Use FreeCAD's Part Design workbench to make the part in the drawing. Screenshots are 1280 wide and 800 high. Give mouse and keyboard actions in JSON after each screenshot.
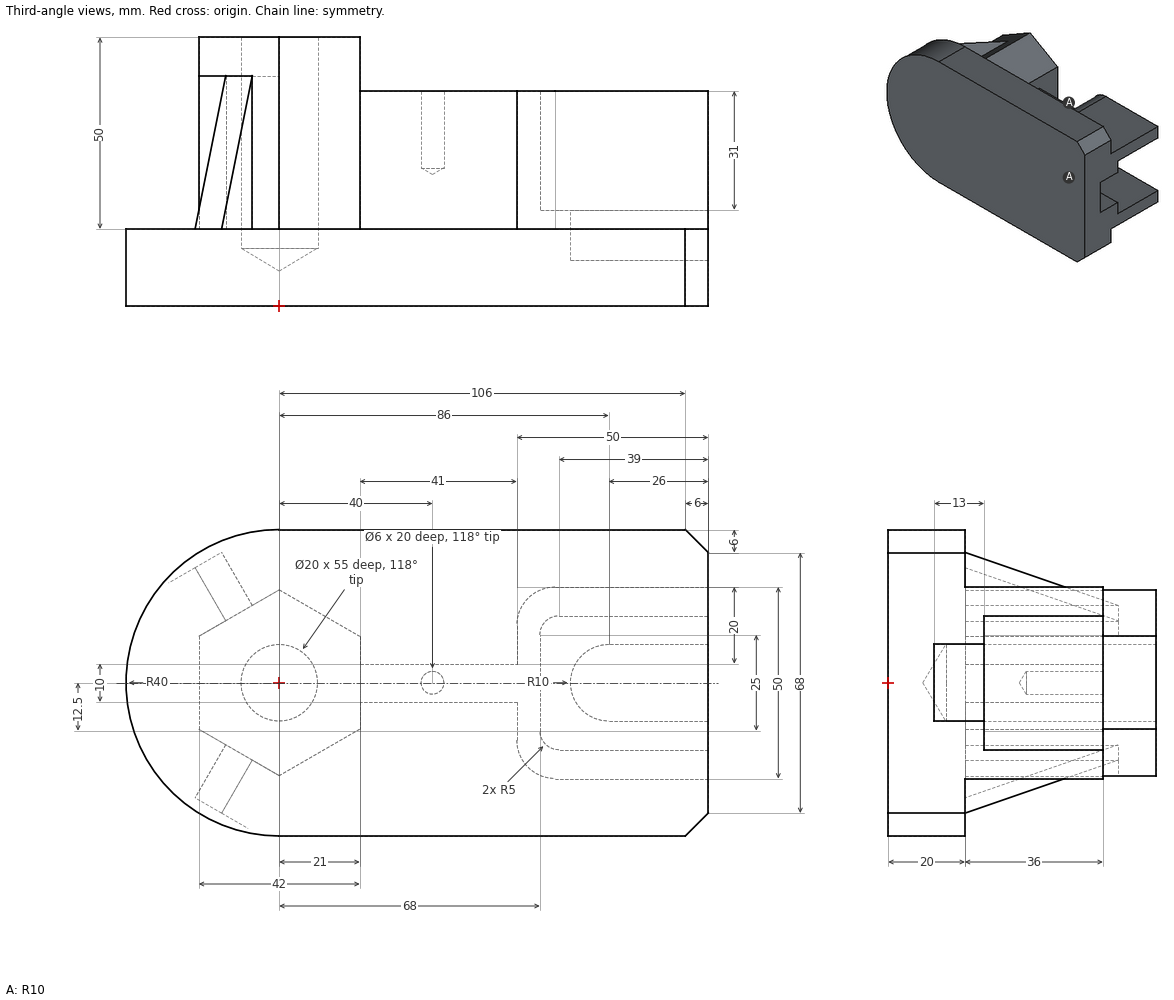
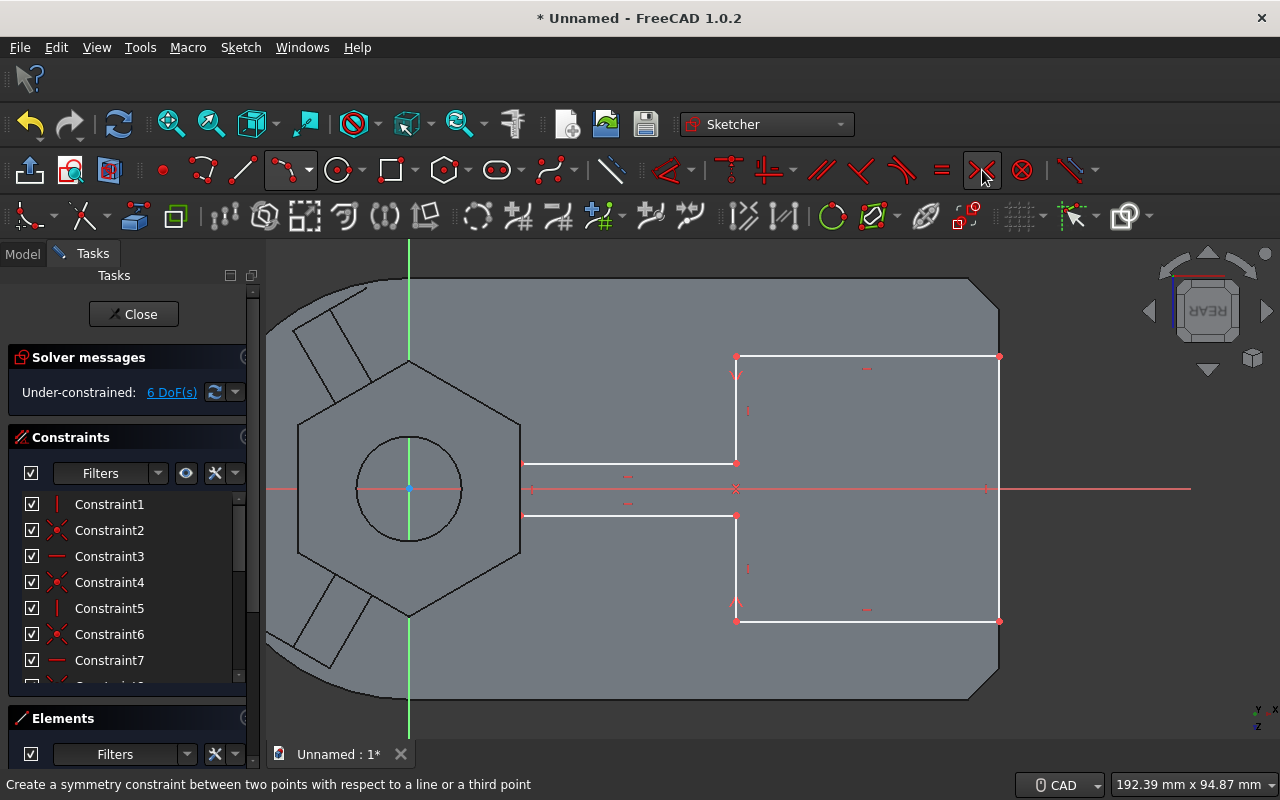
{"action": "left_click", "coordinate": [666, 170]}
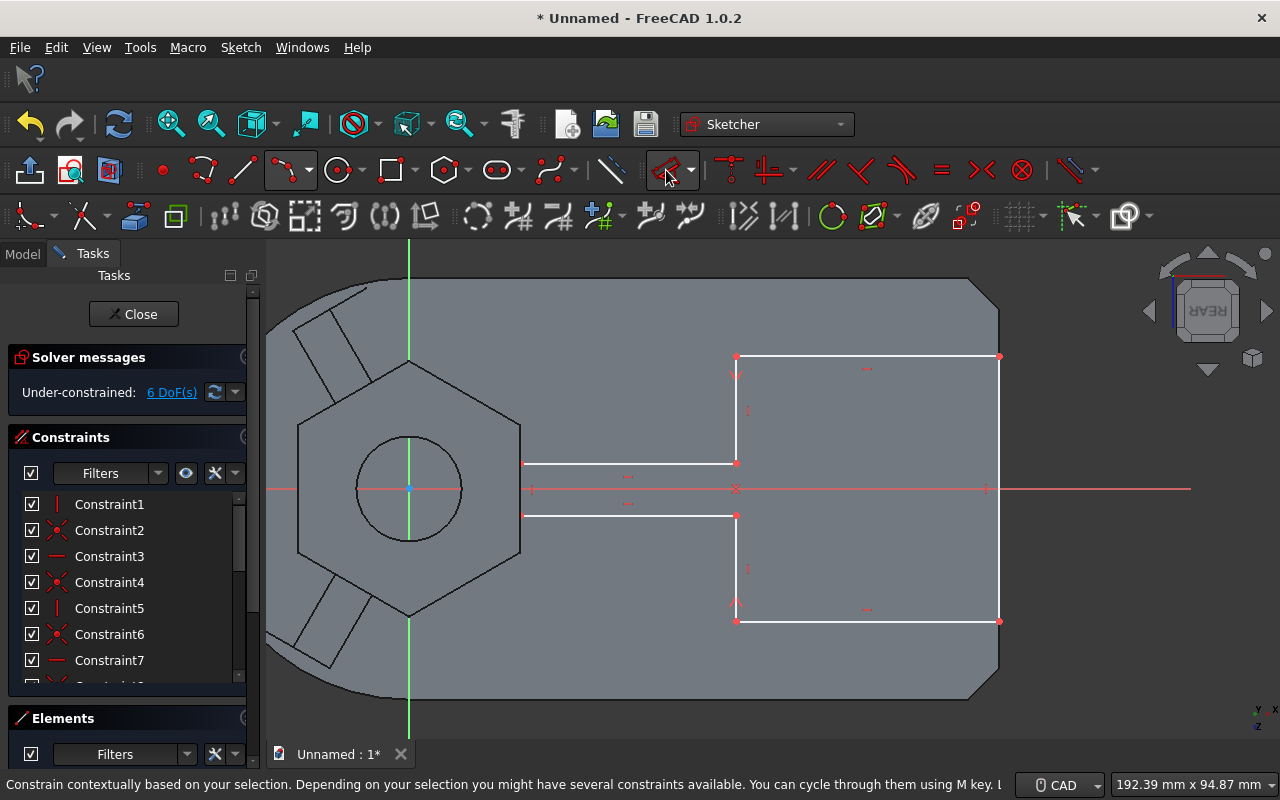
{"action": "scroll", "coordinate": [520, 480], "scroll_direction": "up", "scroll_amount": 2}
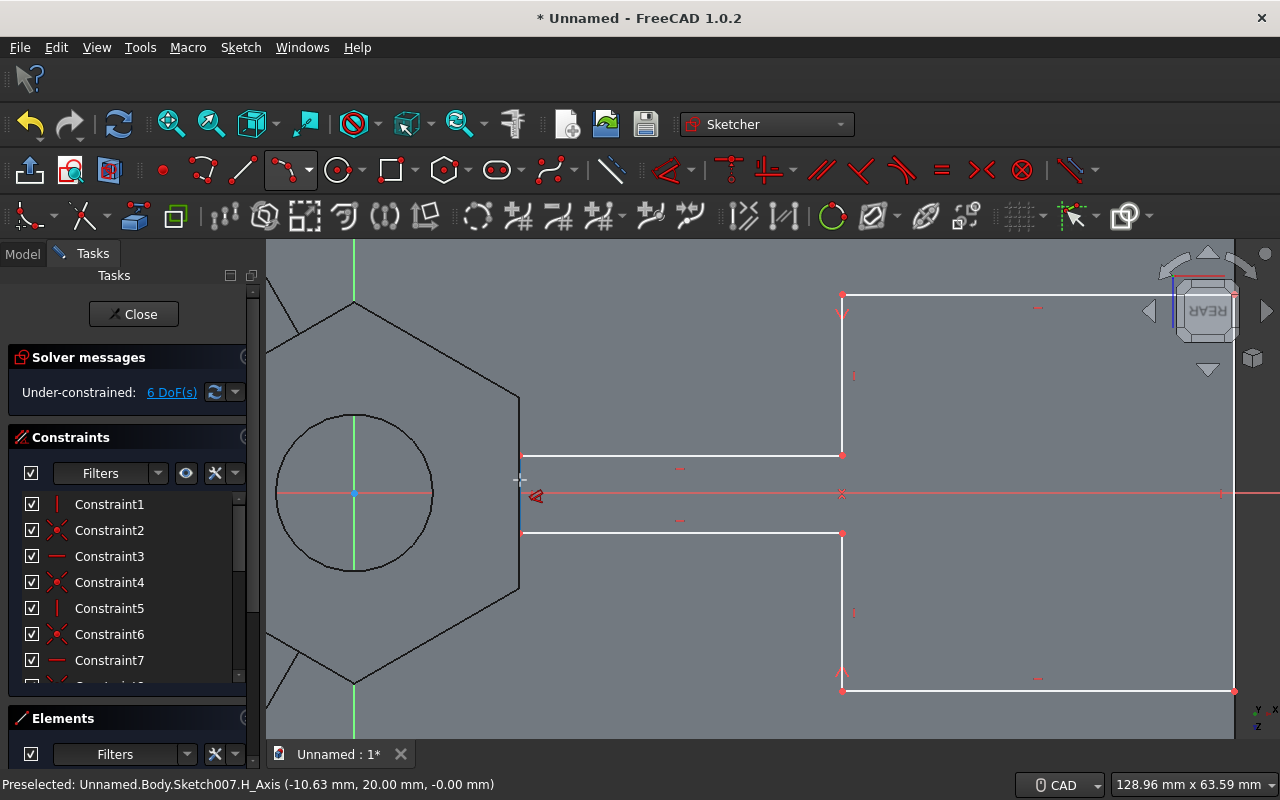
{"action": "left_click", "coordinate": [520, 479]}
{"action": "left_click", "coordinate": [486, 477]}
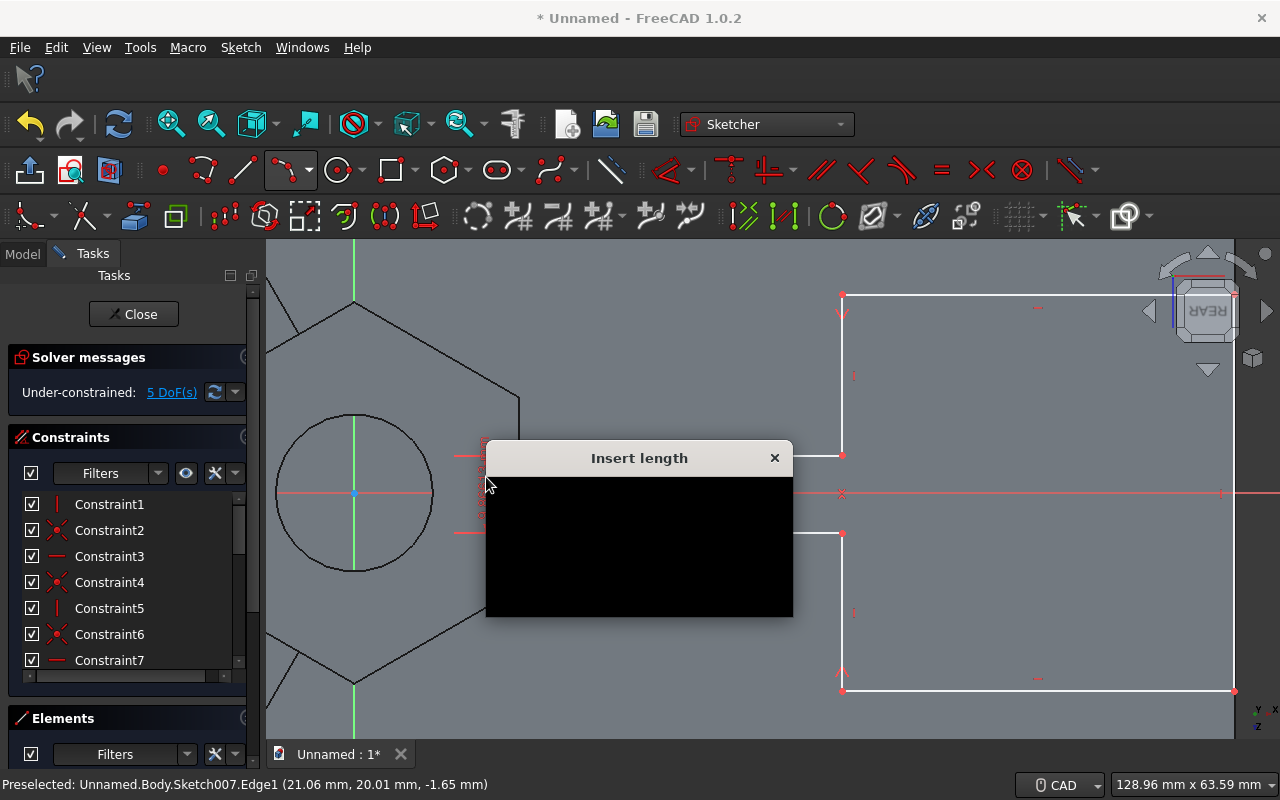
{"action": "type", "text": "10"}
{"action": "key", "text": "Return"}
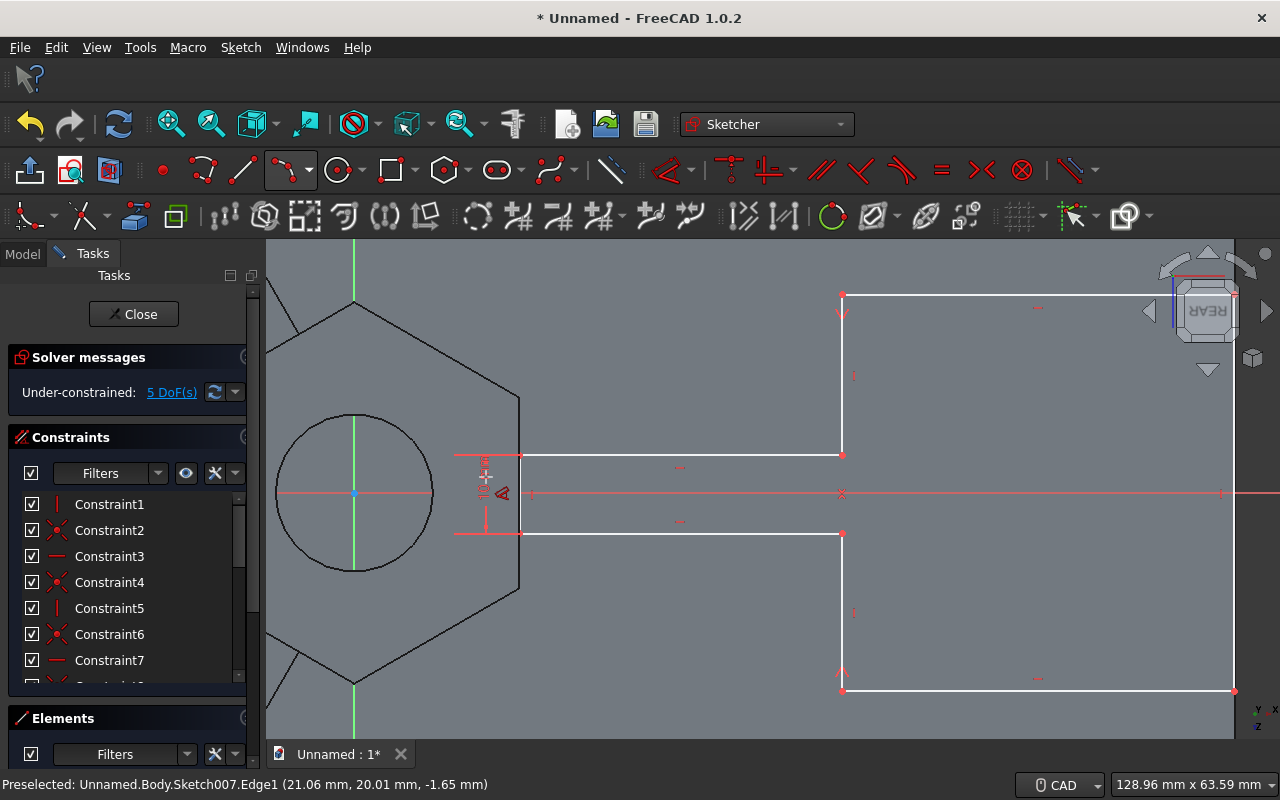
{"action": "left_click", "coordinate": [617, 534]}
{"action": "left_click", "coordinate": [681, 568]}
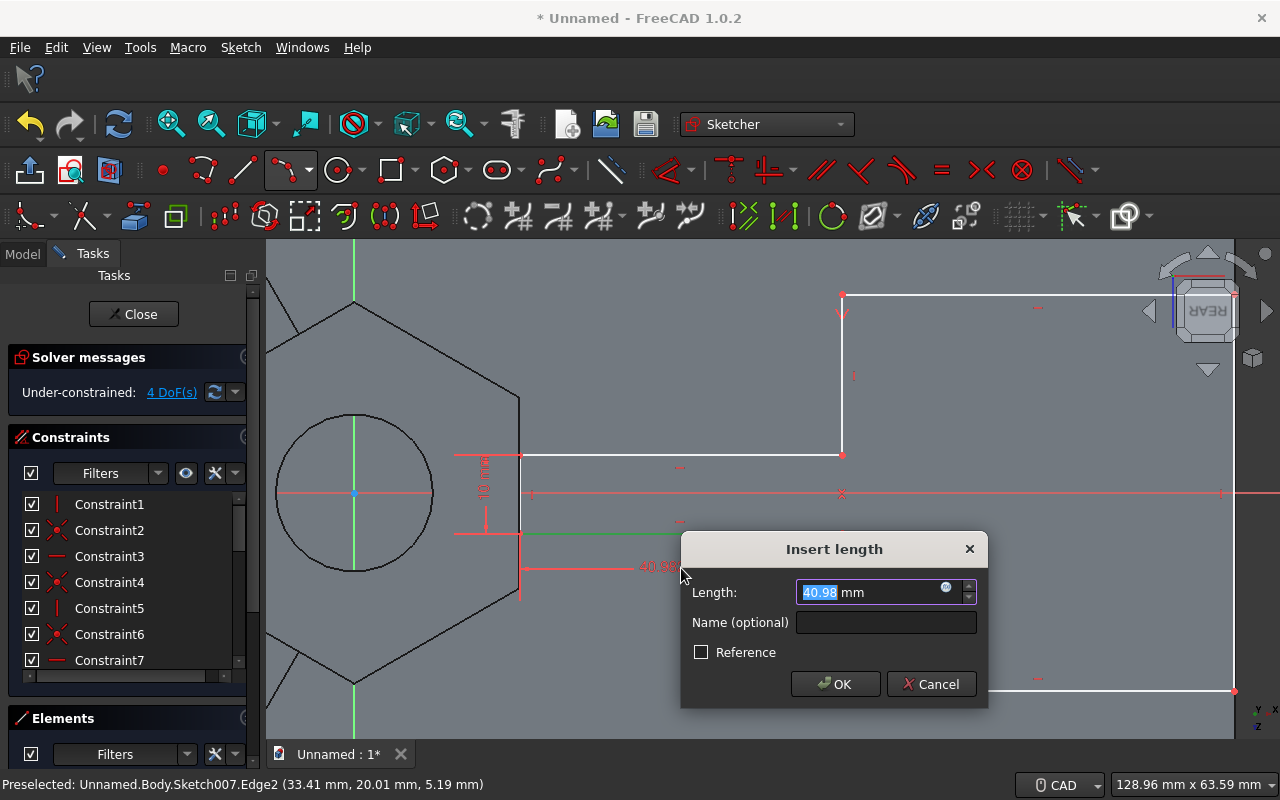
{"action": "type", "text": "41"}
{"action": "key", "text": "Return"}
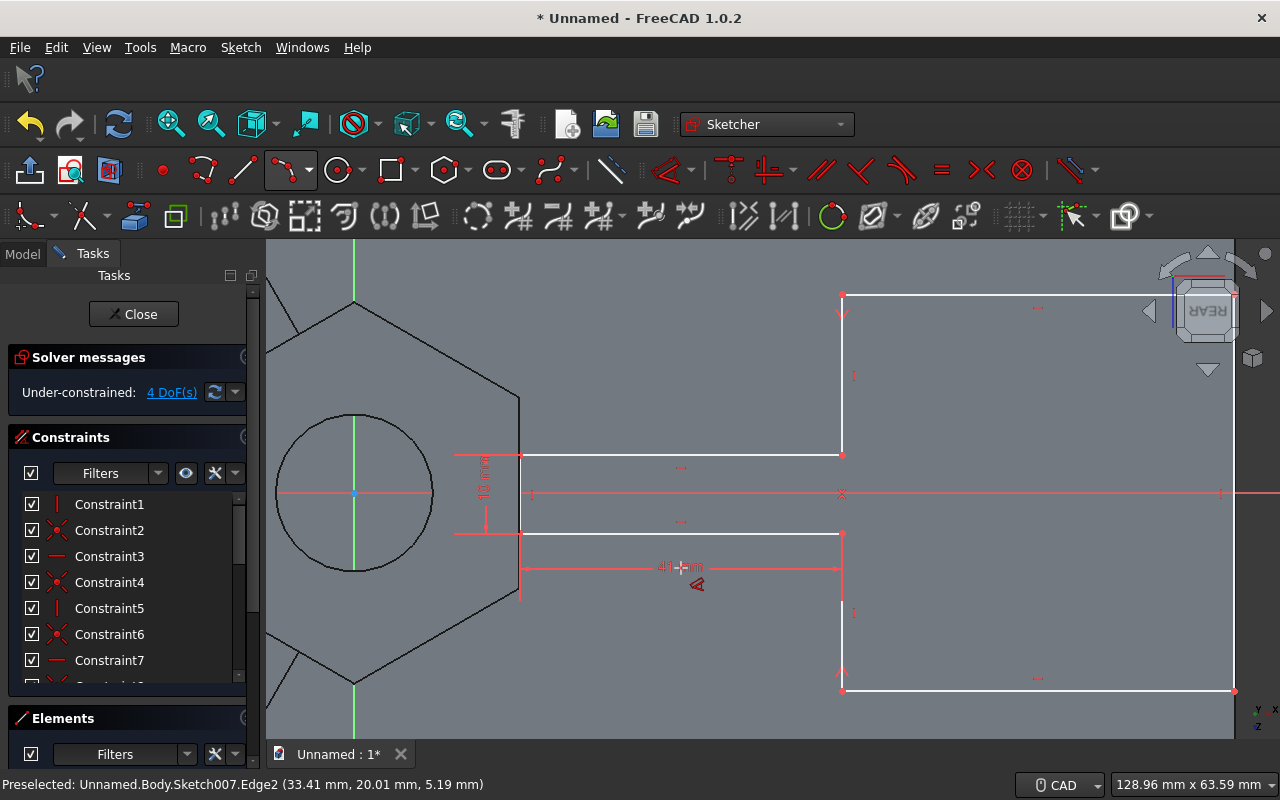
{"action": "left_click", "coordinate": [842, 581]}
{"action": "left_click", "coordinate": [876, 612]}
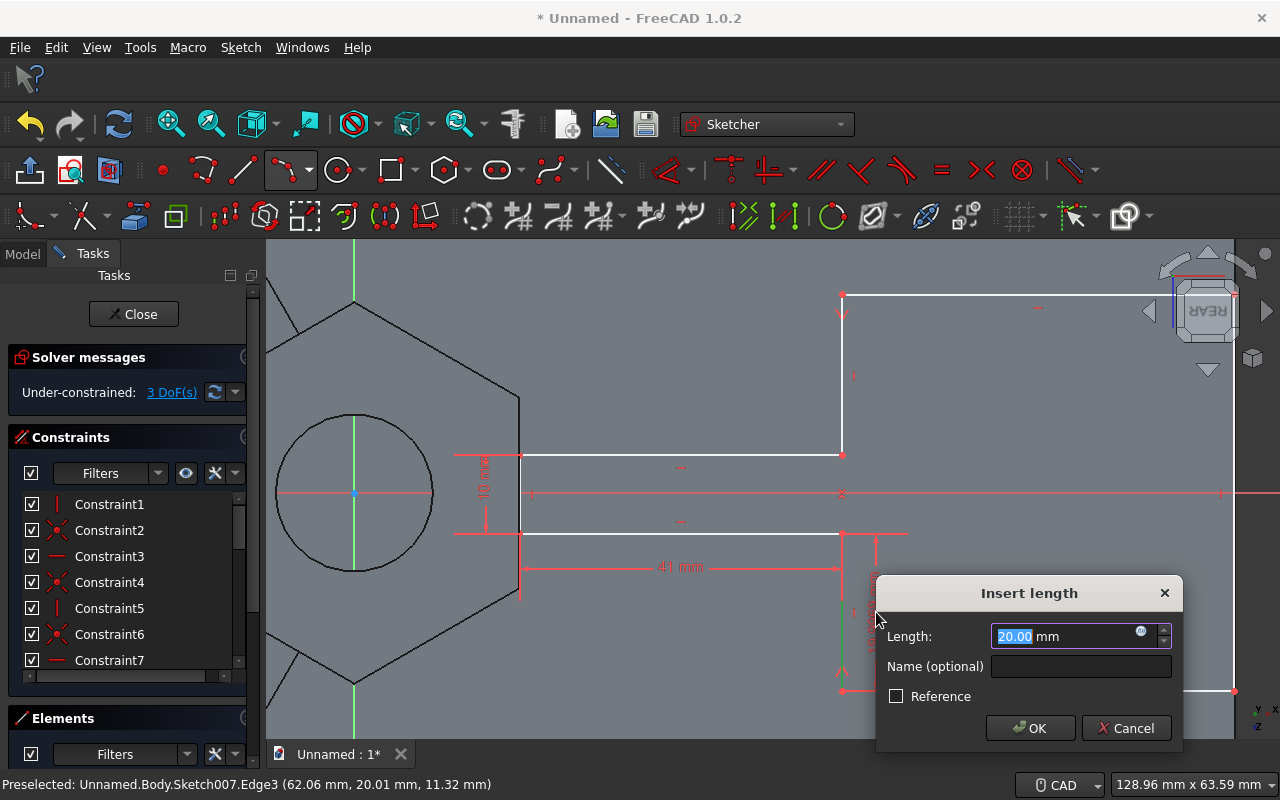
{"action": "type", "text": "20"}
{"action": "key", "text": "Return"}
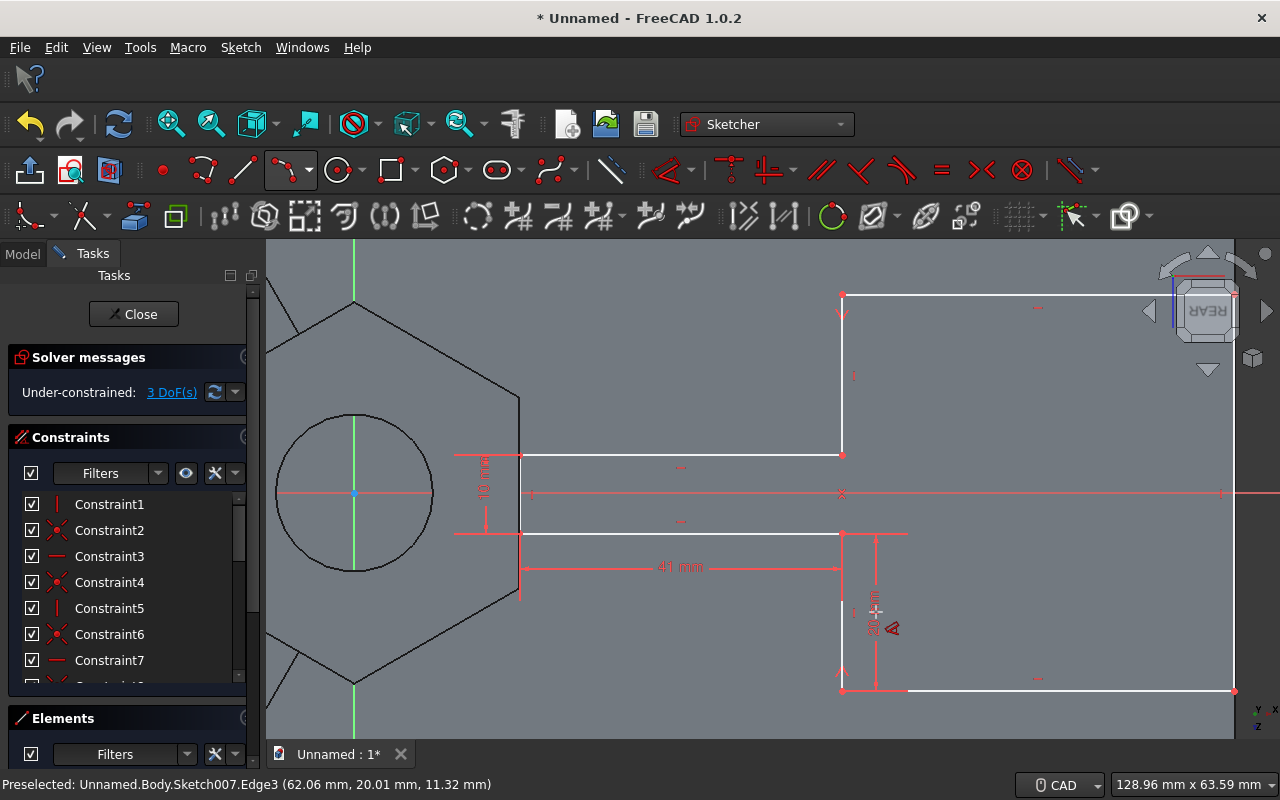
{"action": "left_click", "coordinate": [960, 691]}
{"action": "left_click", "coordinate": [979, 657]}